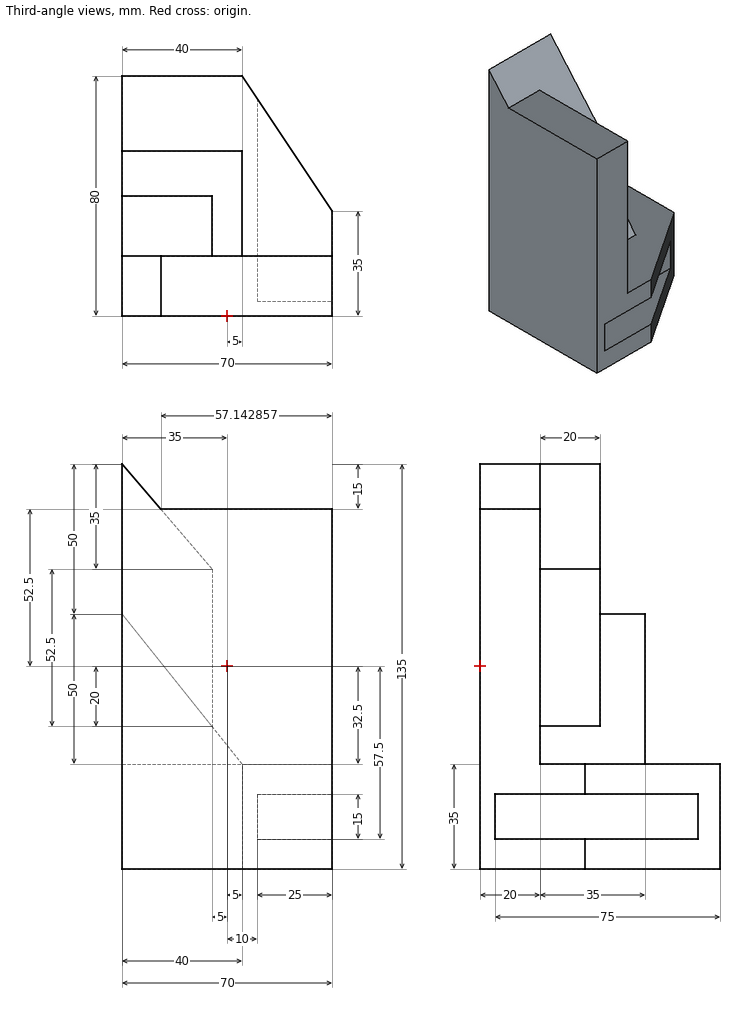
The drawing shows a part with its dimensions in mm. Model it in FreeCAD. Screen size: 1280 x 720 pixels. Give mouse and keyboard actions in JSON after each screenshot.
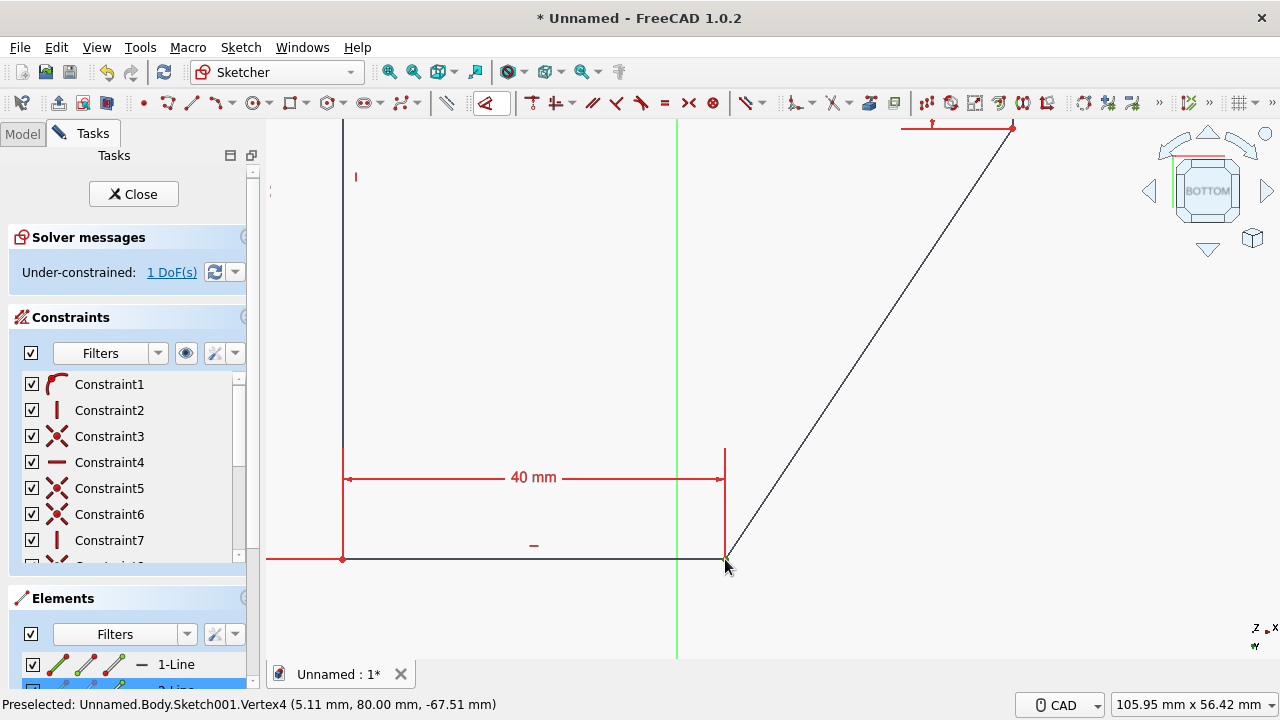
{"action": "left_click", "coordinate": [504, 104]}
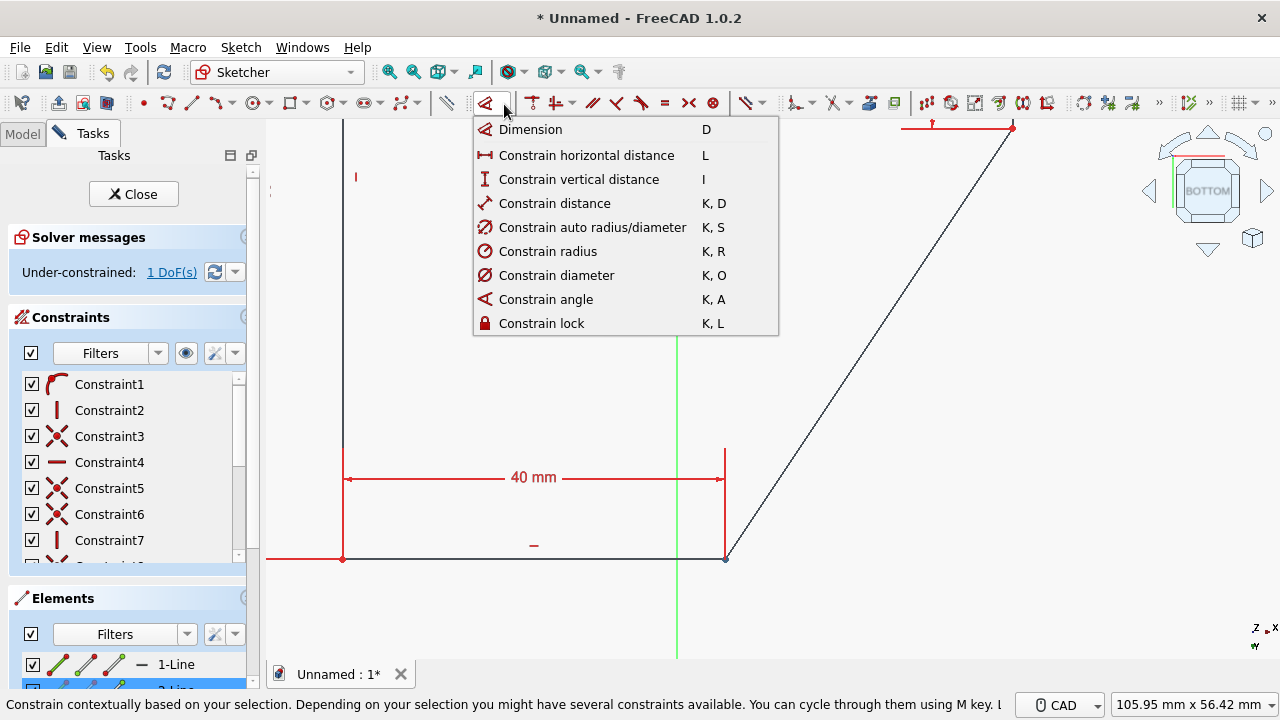
{"action": "left_click", "coordinate": [626, 155]}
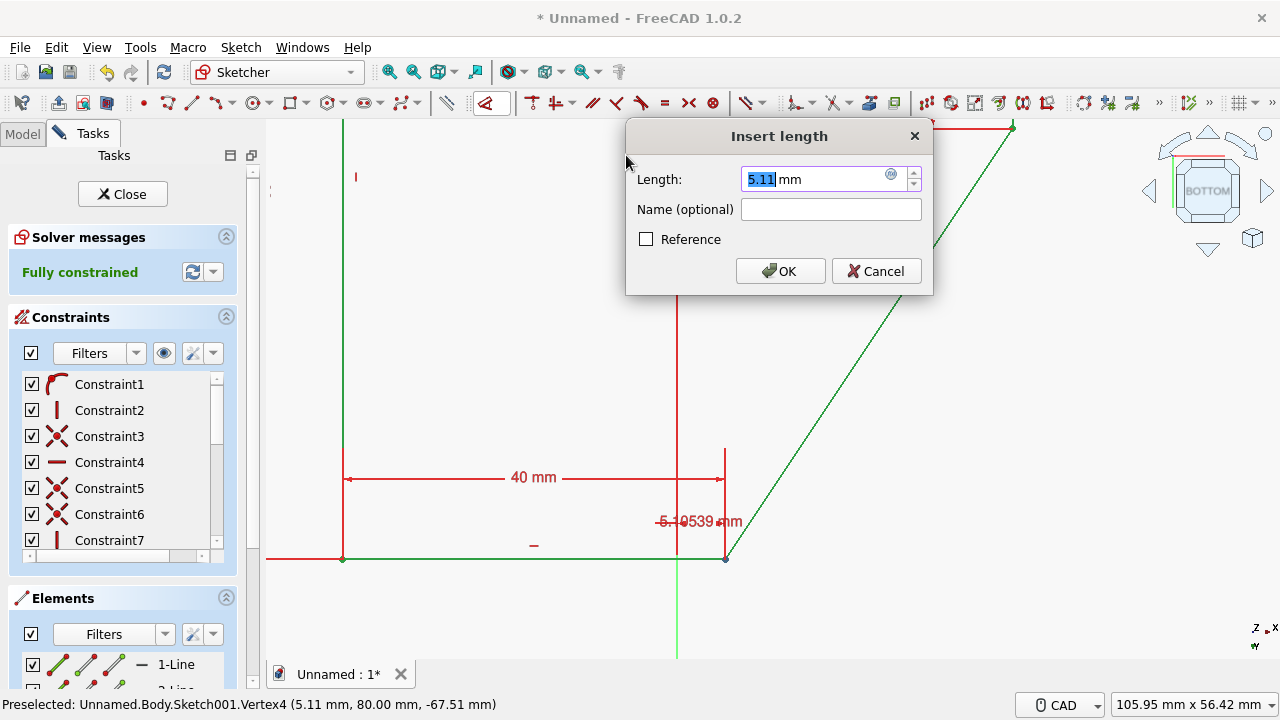
{"action": "type", "text": "5"}
{"action": "key", "text": "Return"}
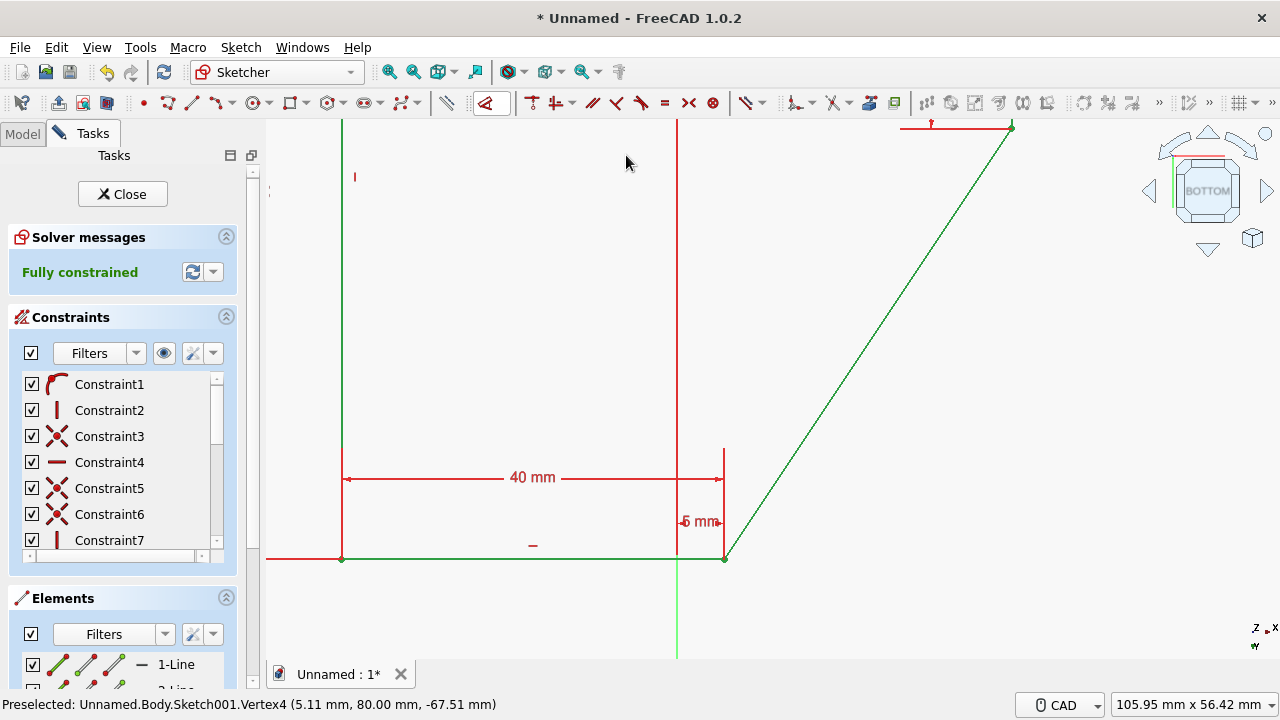
{"action": "left_click", "coordinate": [123, 194]}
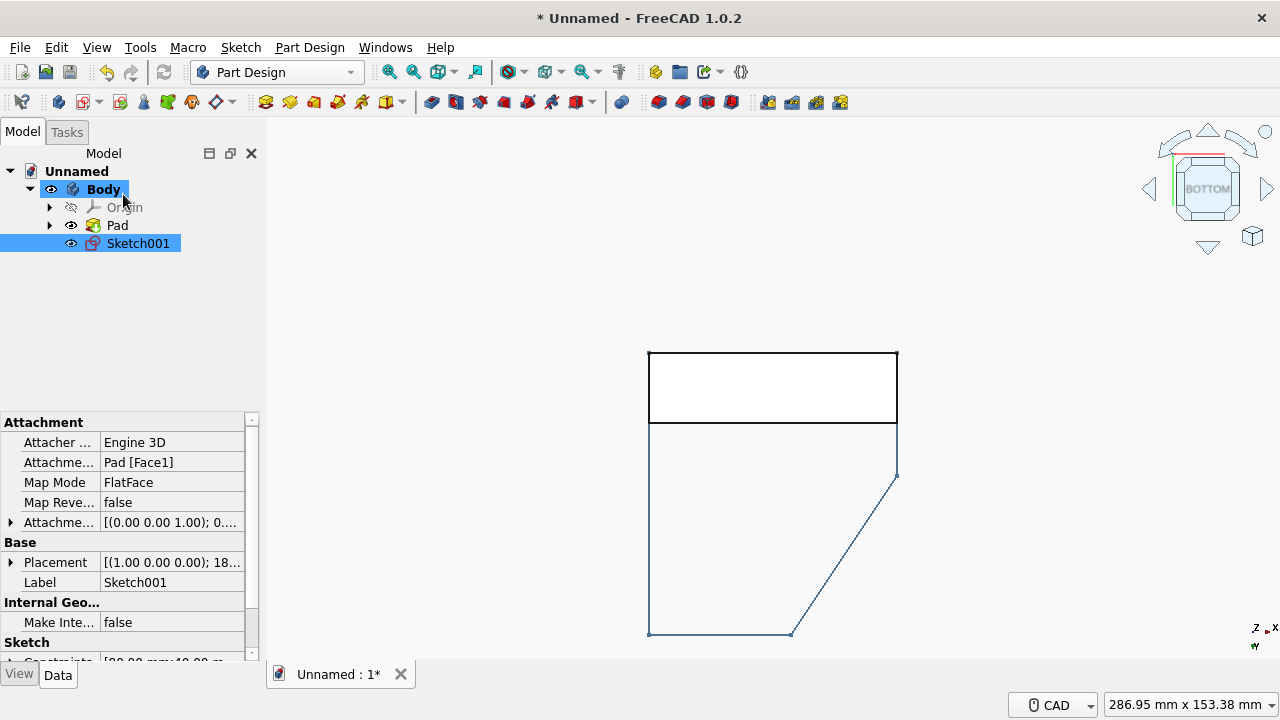
{"action": "left_click", "coordinate": [266, 102]}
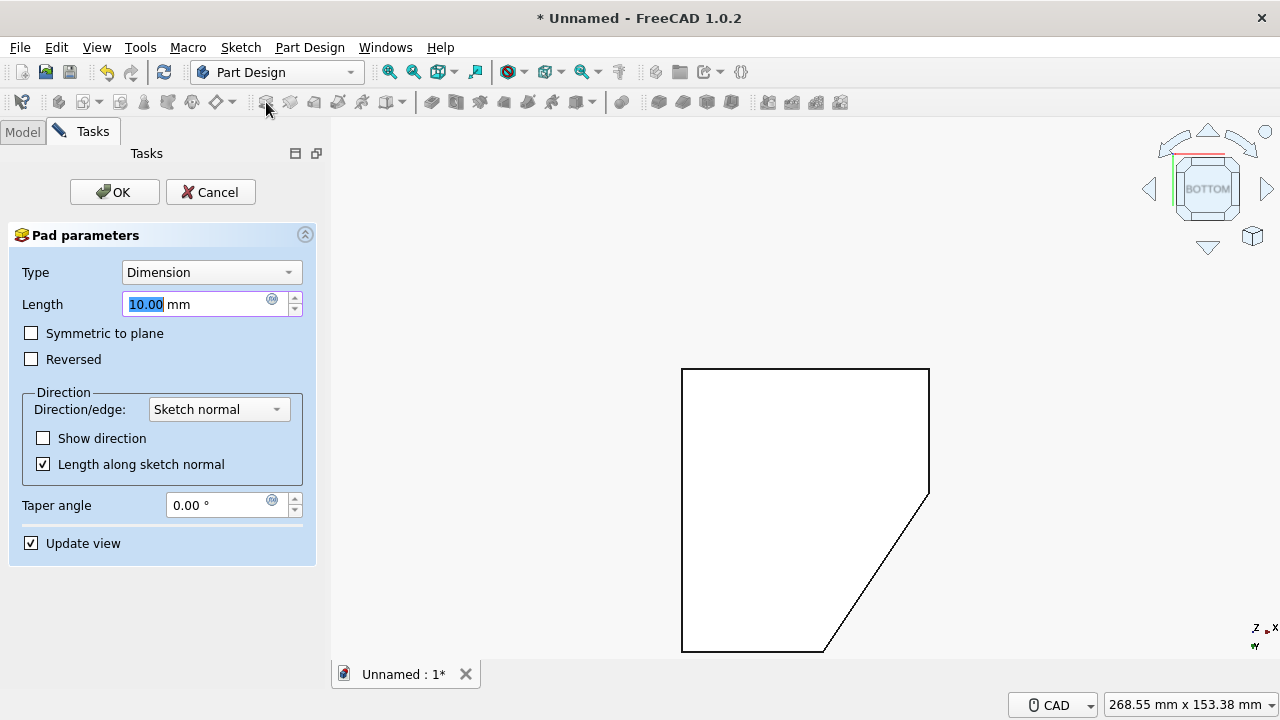
{"action": "type", "text": "35"}
{"action": "key", "text": "Tab"}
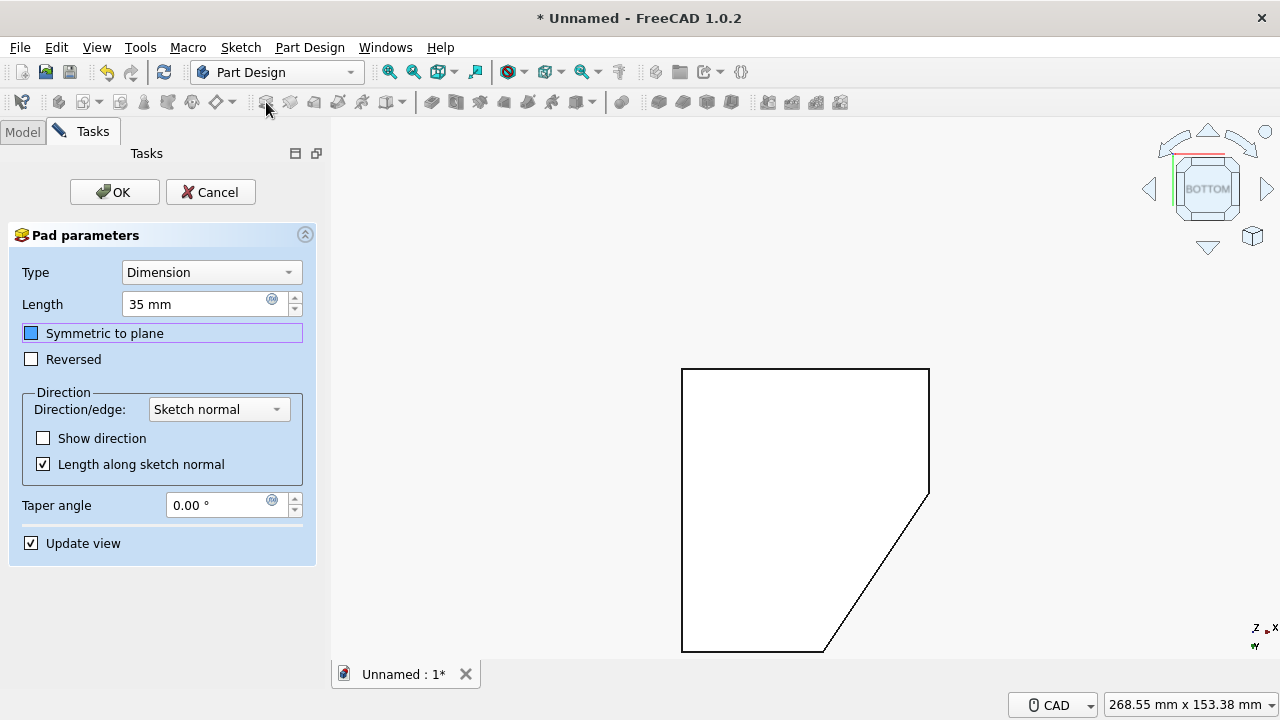
{"action": "left_click", "coordinate": [30, 359]}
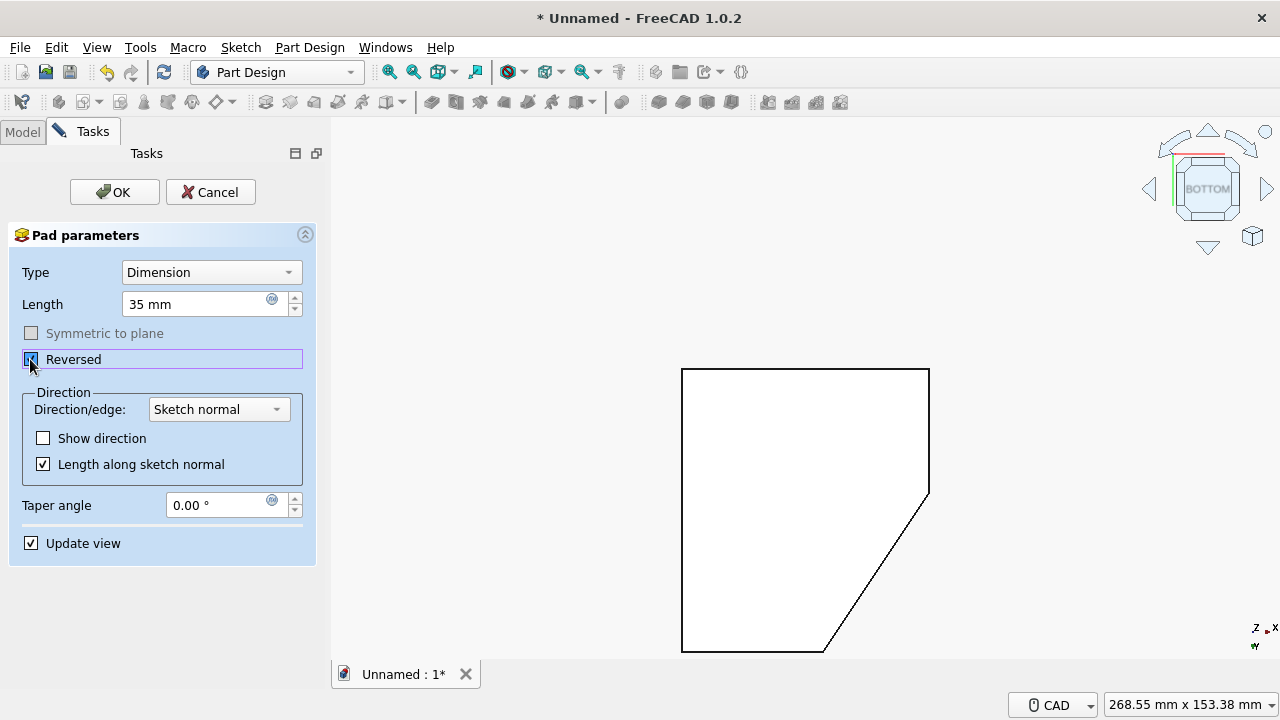
{"action": "left_click", "coordinate": [115, 192]}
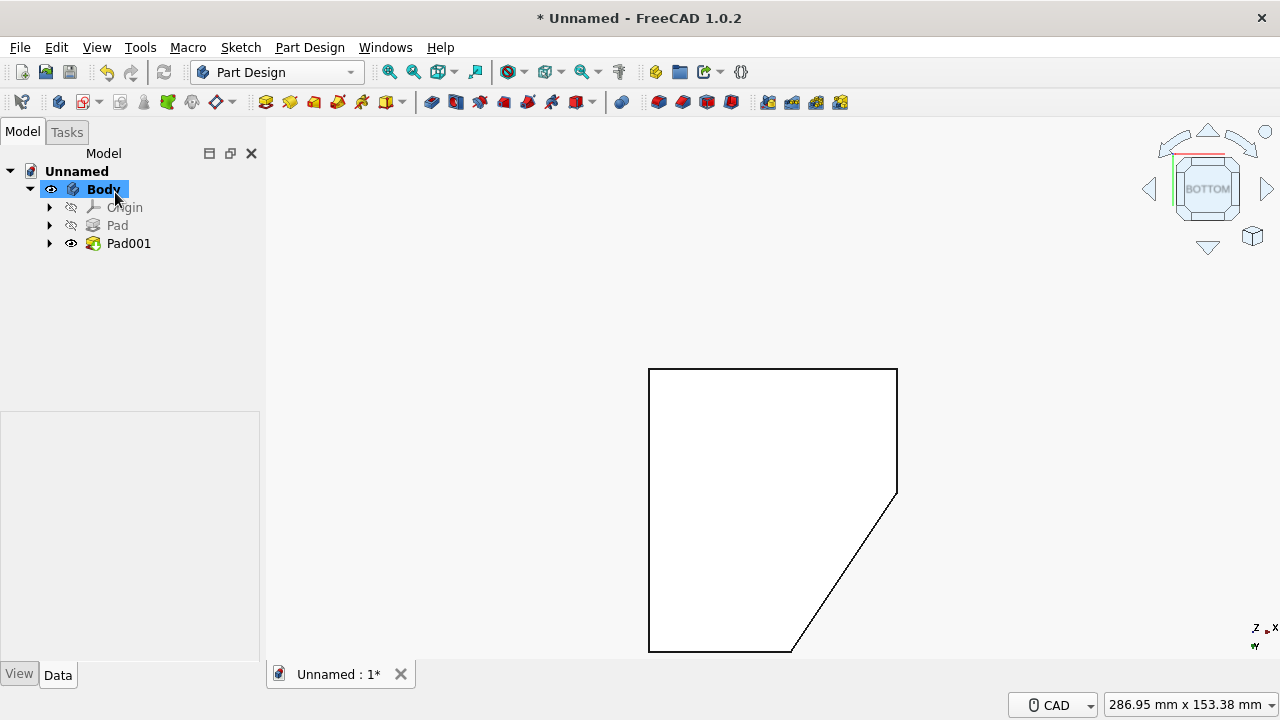
{"action": "key", "text": "4"}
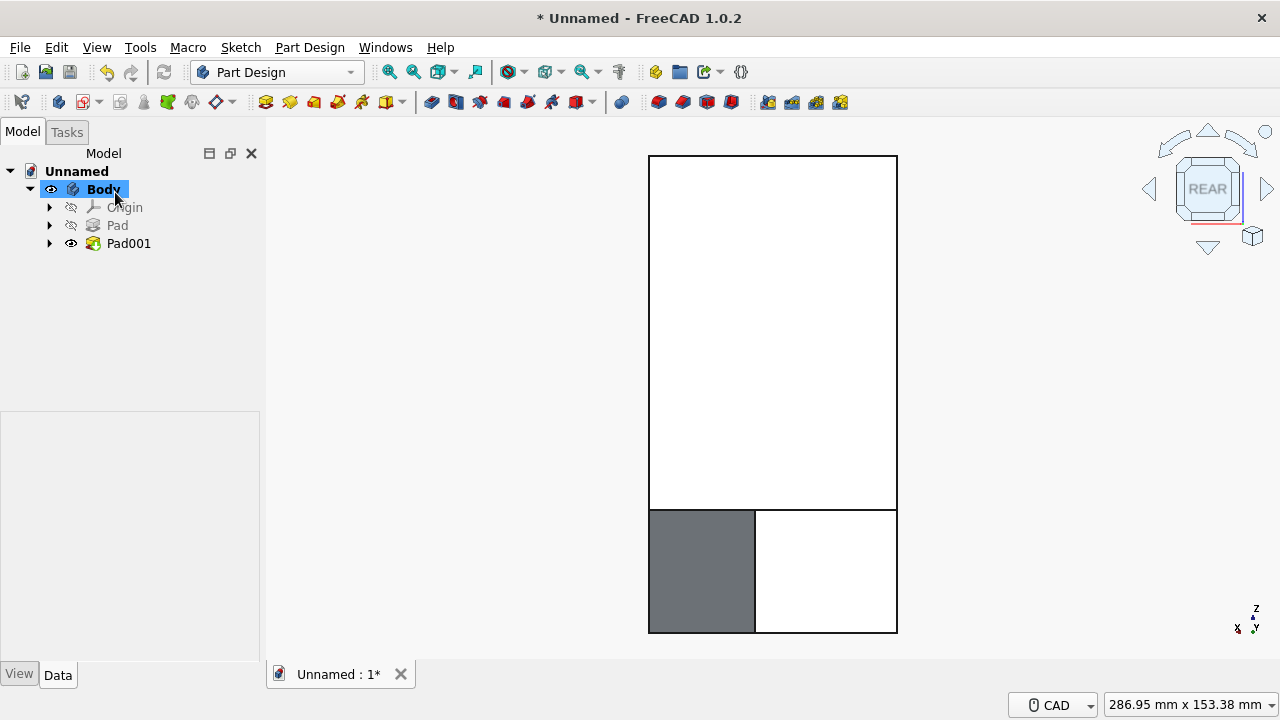
{"action": "left_click", "coordinate": [826, 571]}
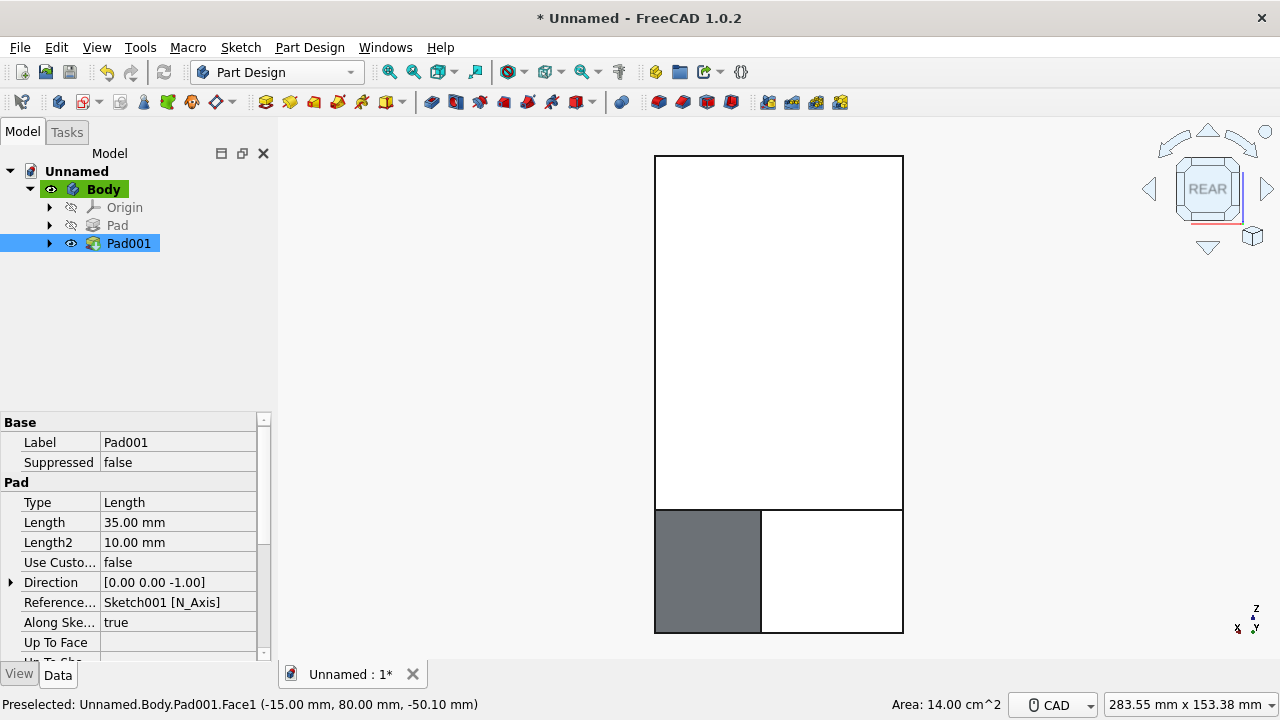
{"action": "left_click", "coordinate": [84, 102]}